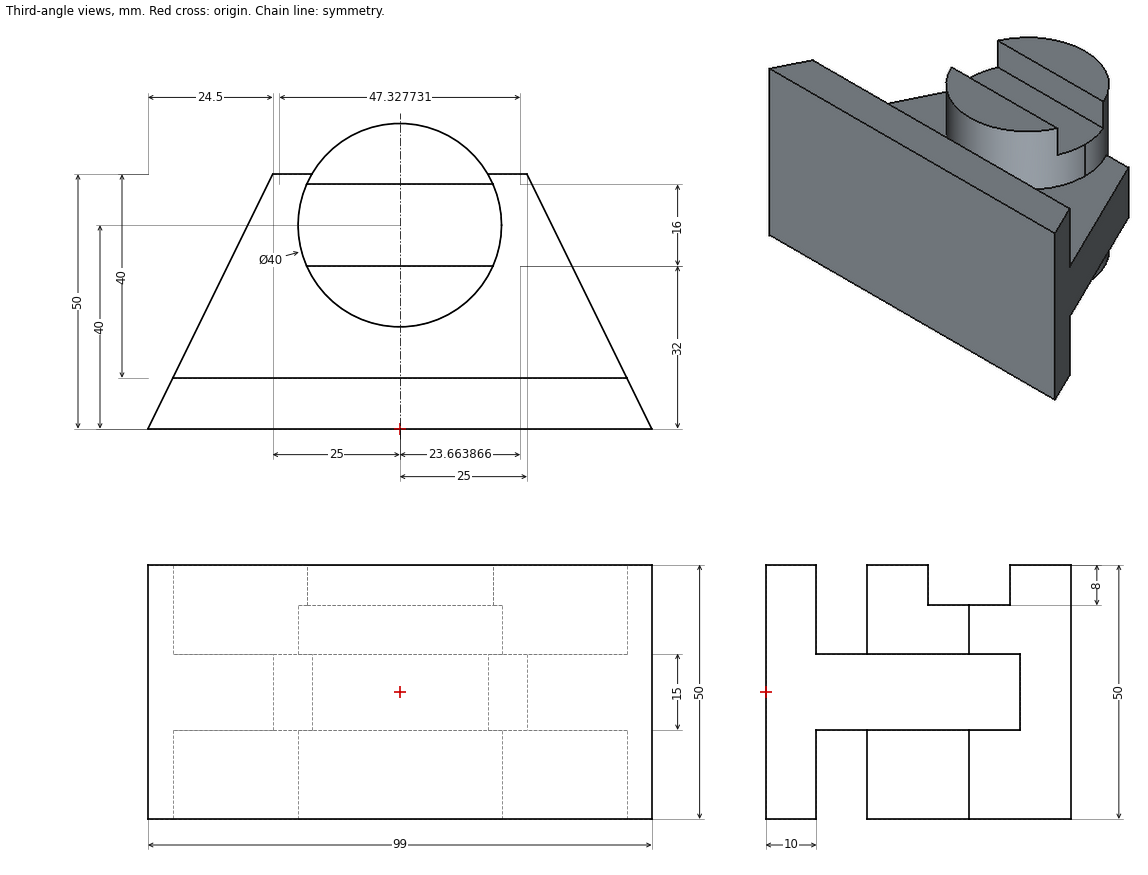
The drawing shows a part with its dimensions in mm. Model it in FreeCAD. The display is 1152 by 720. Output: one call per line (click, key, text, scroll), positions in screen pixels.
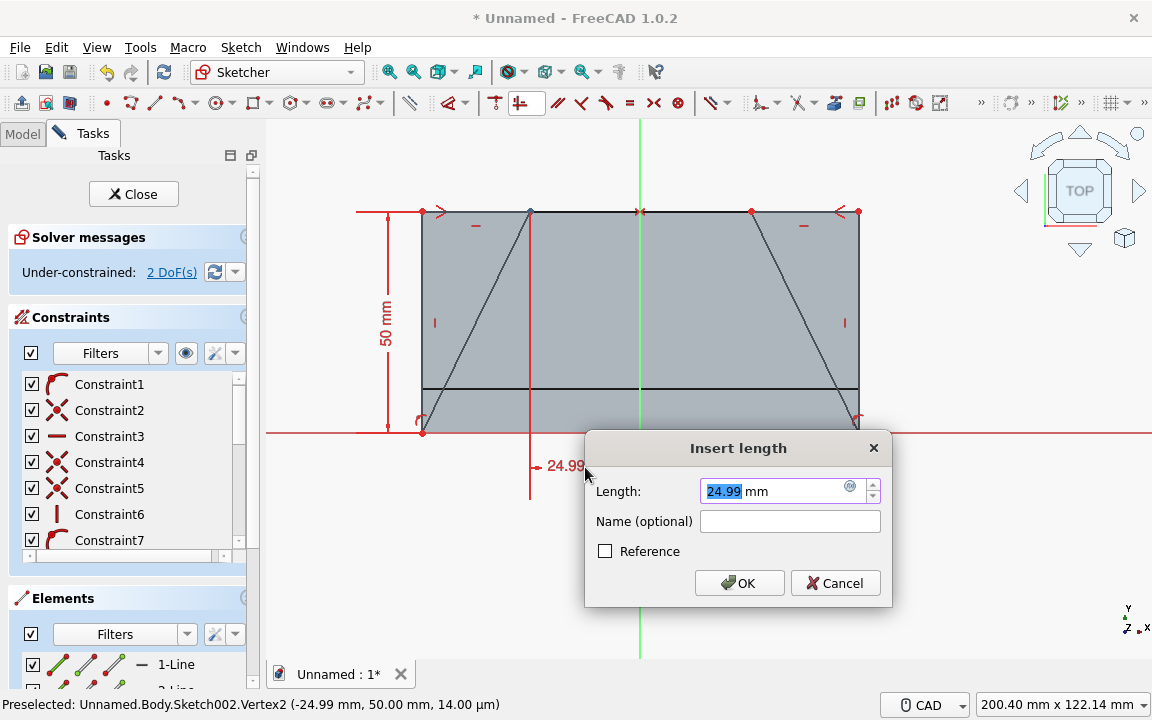
text(25)
key(Return)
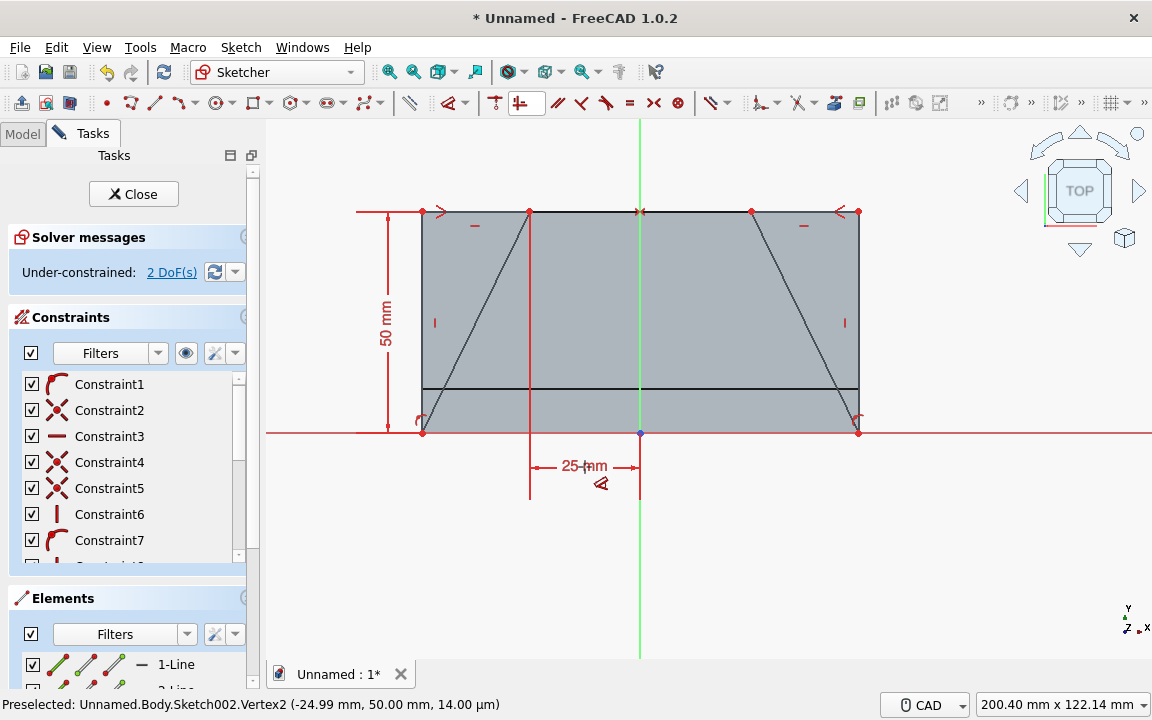
click(751, 212)
click(696, 467)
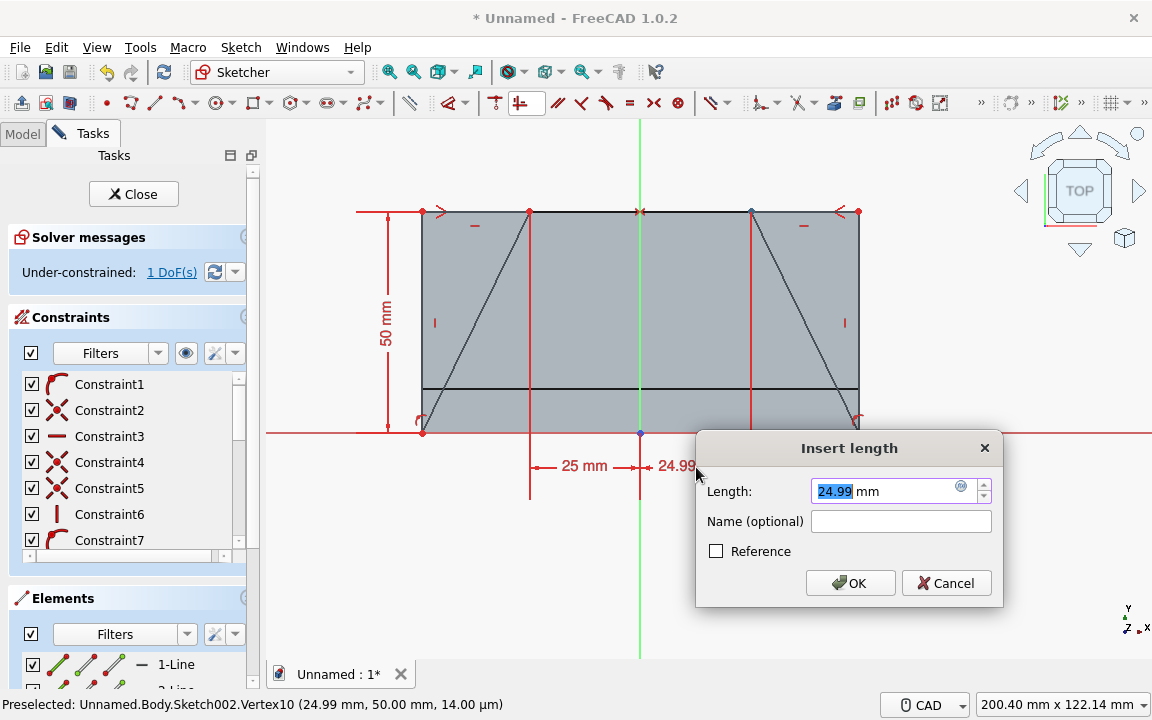
text(25)
key(Return)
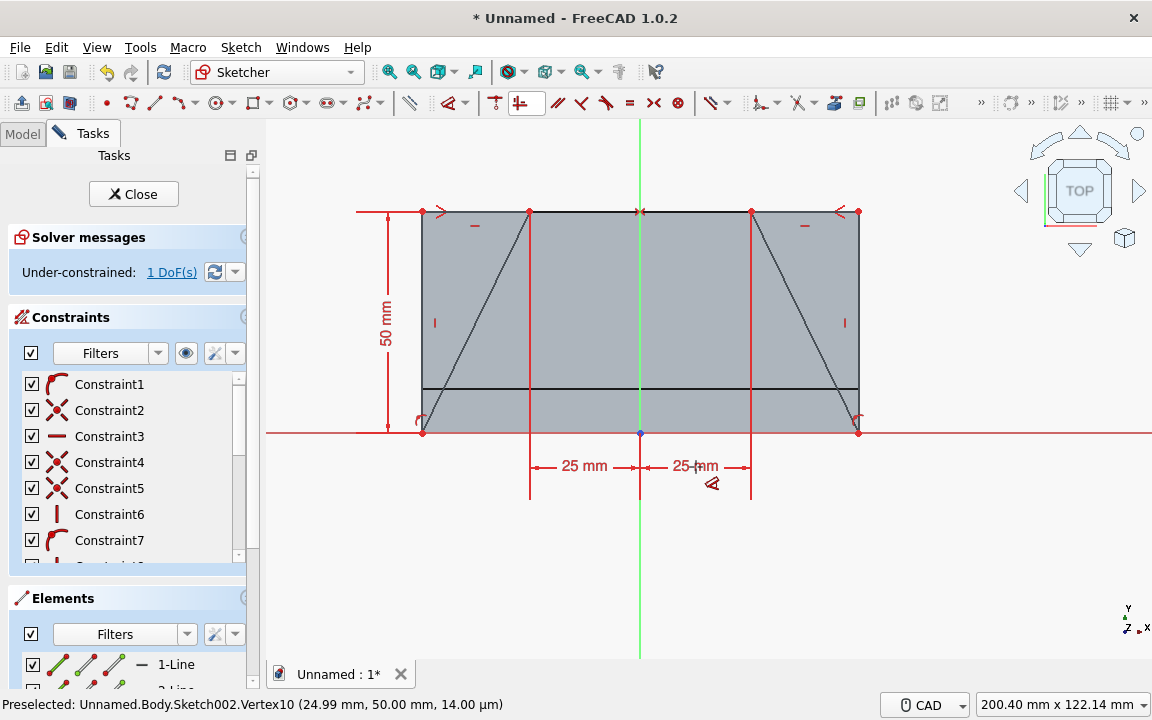
click(498, 212)
click(476, 178)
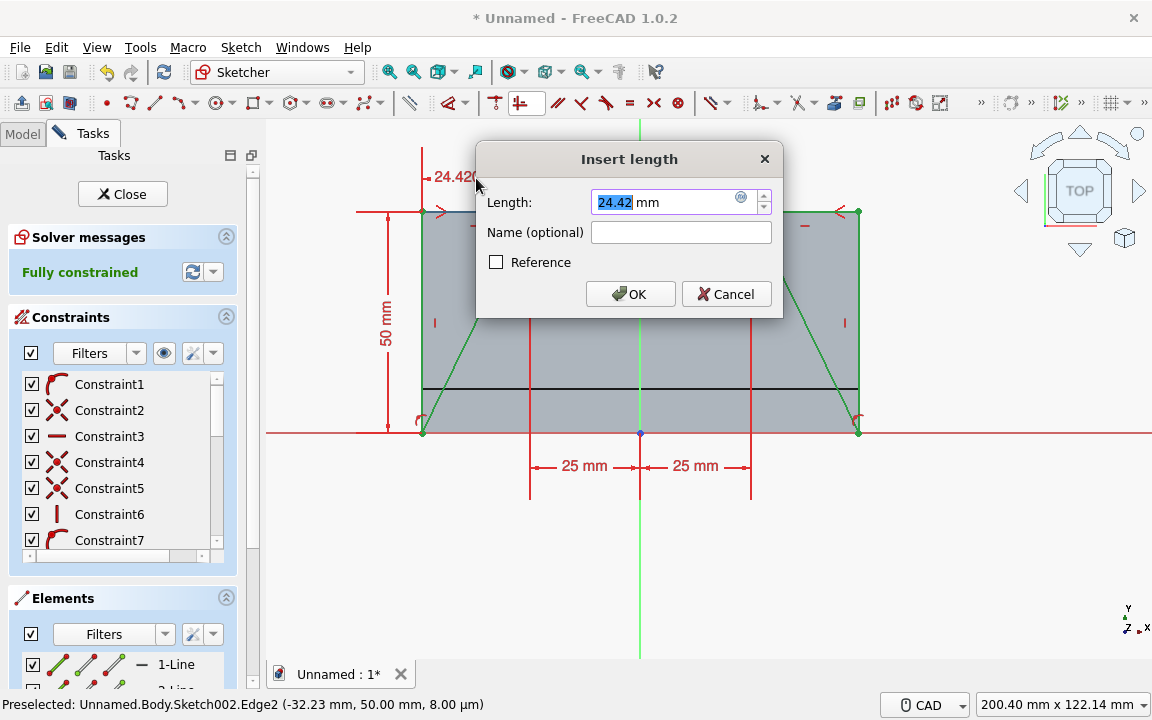
text(24.5)
key(Return)
key(Escape)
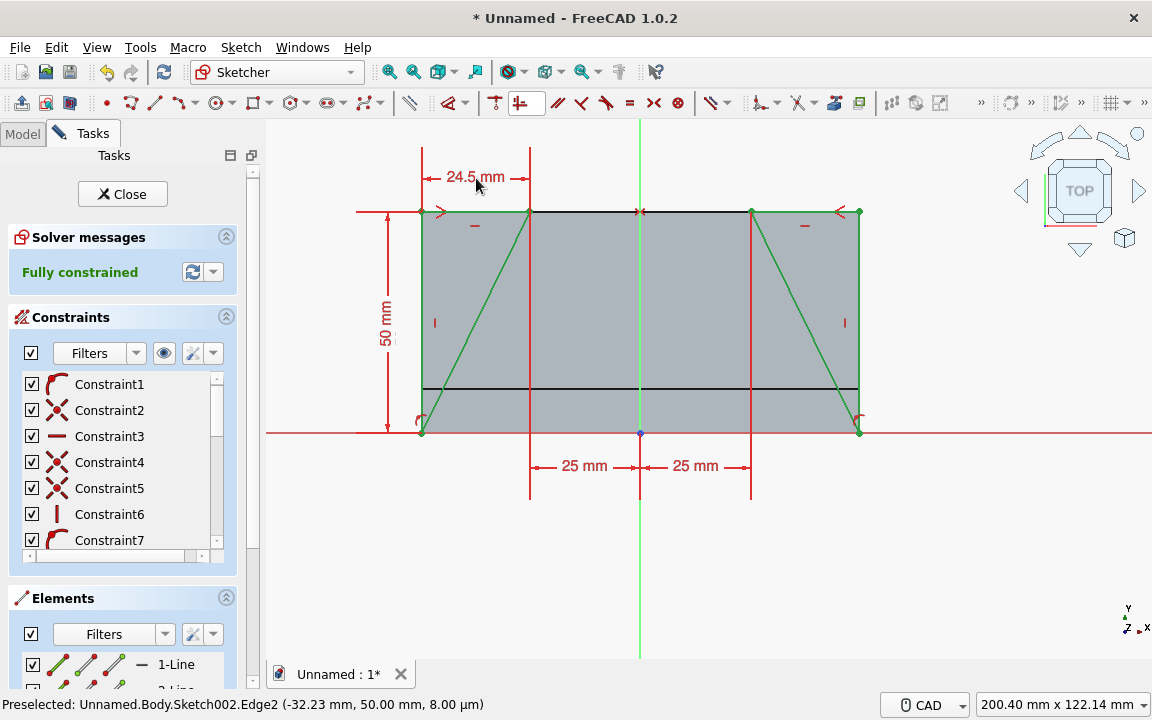
click(123, 194)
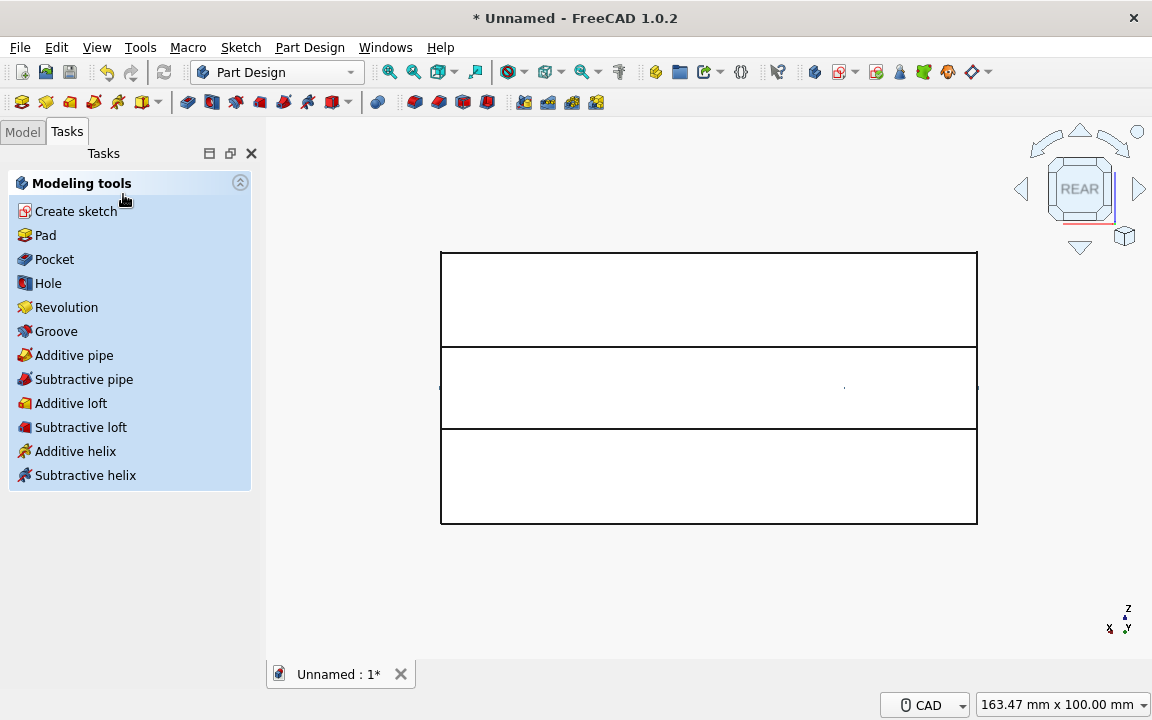
click(188, 102)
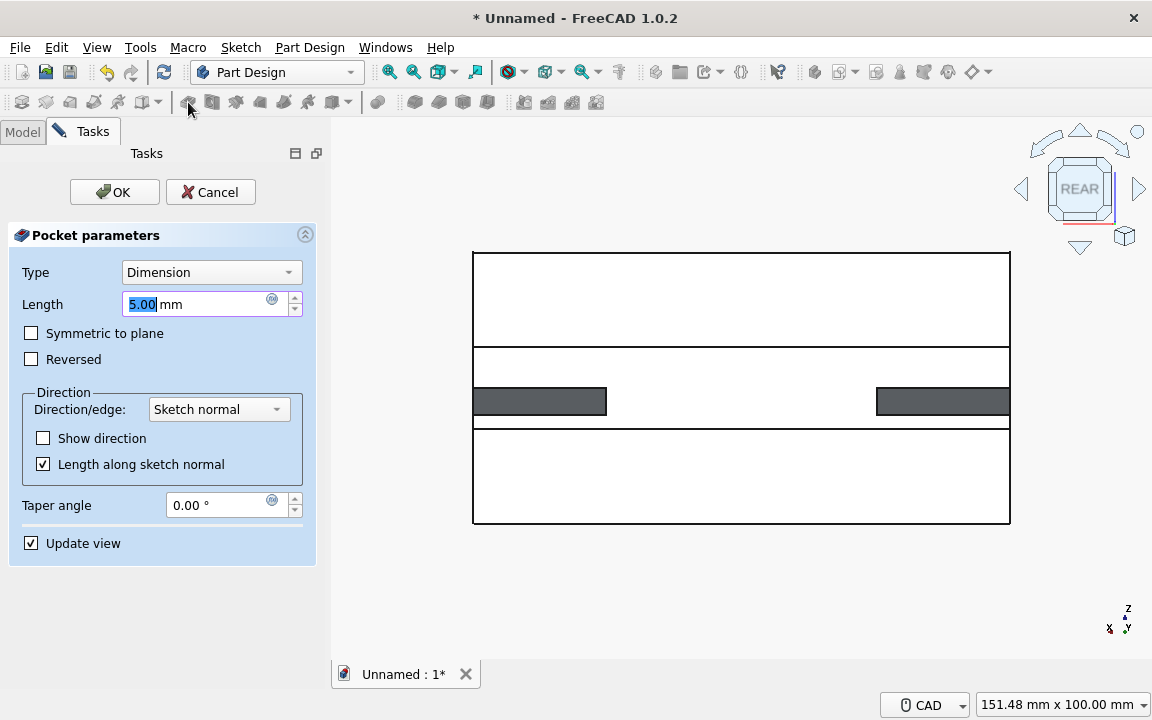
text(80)
key(Tab)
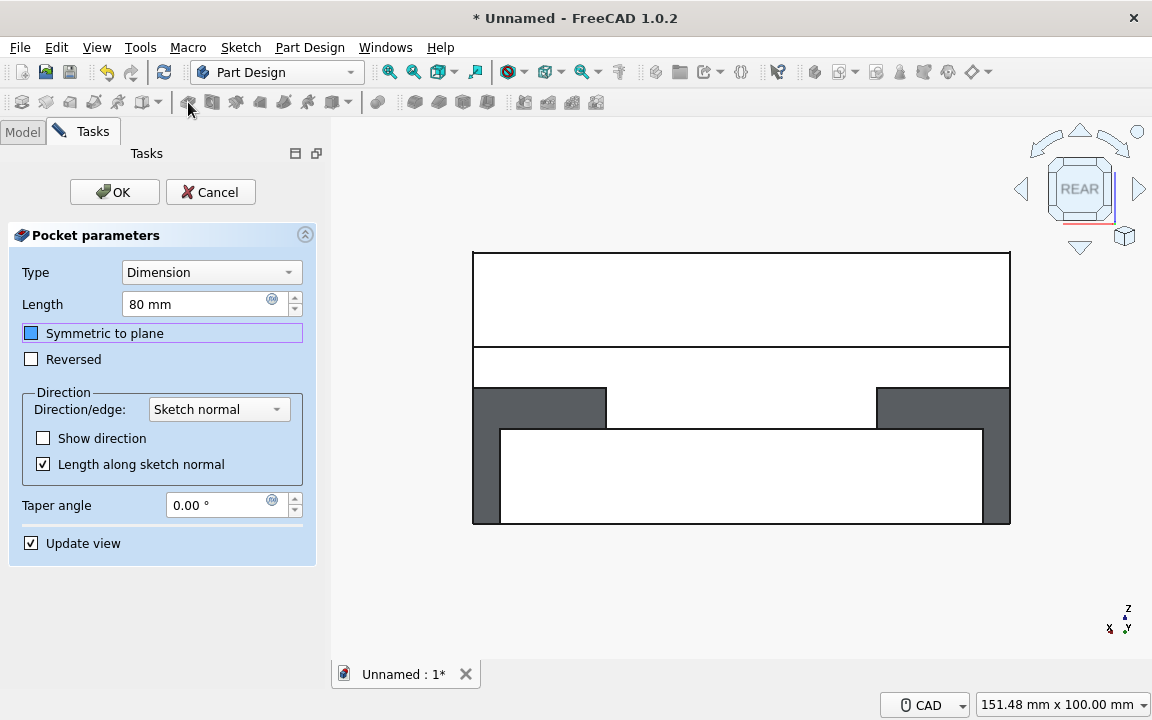
click(30, 333)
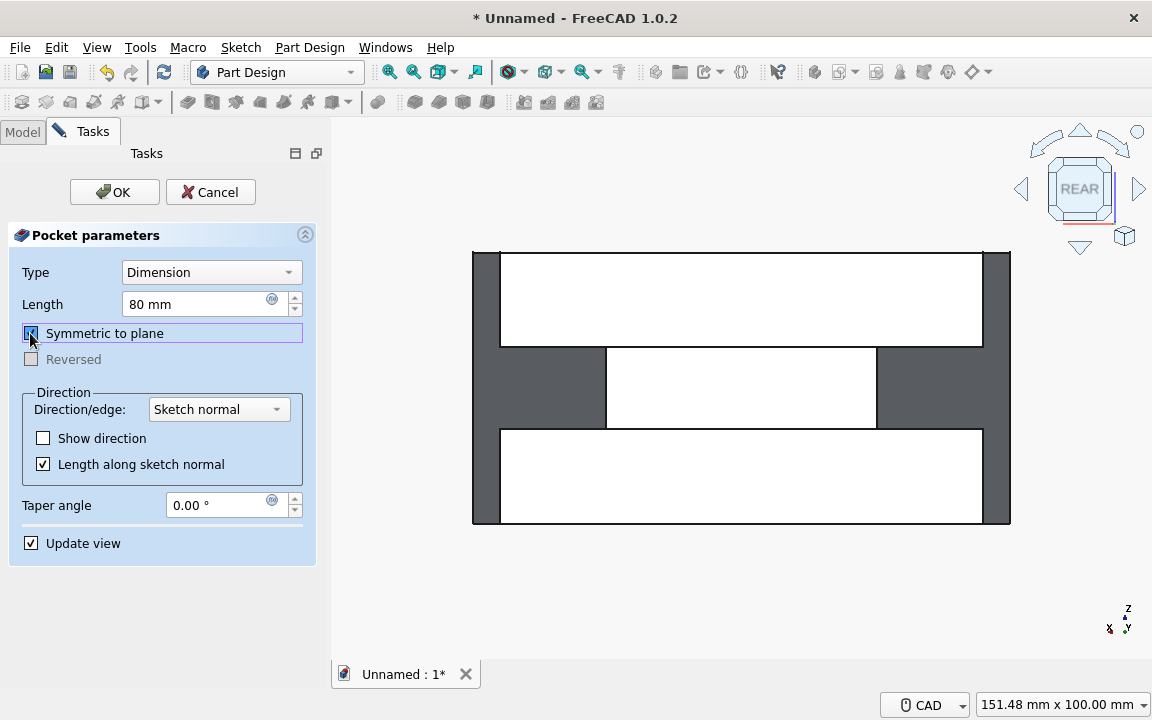
click(115, 192)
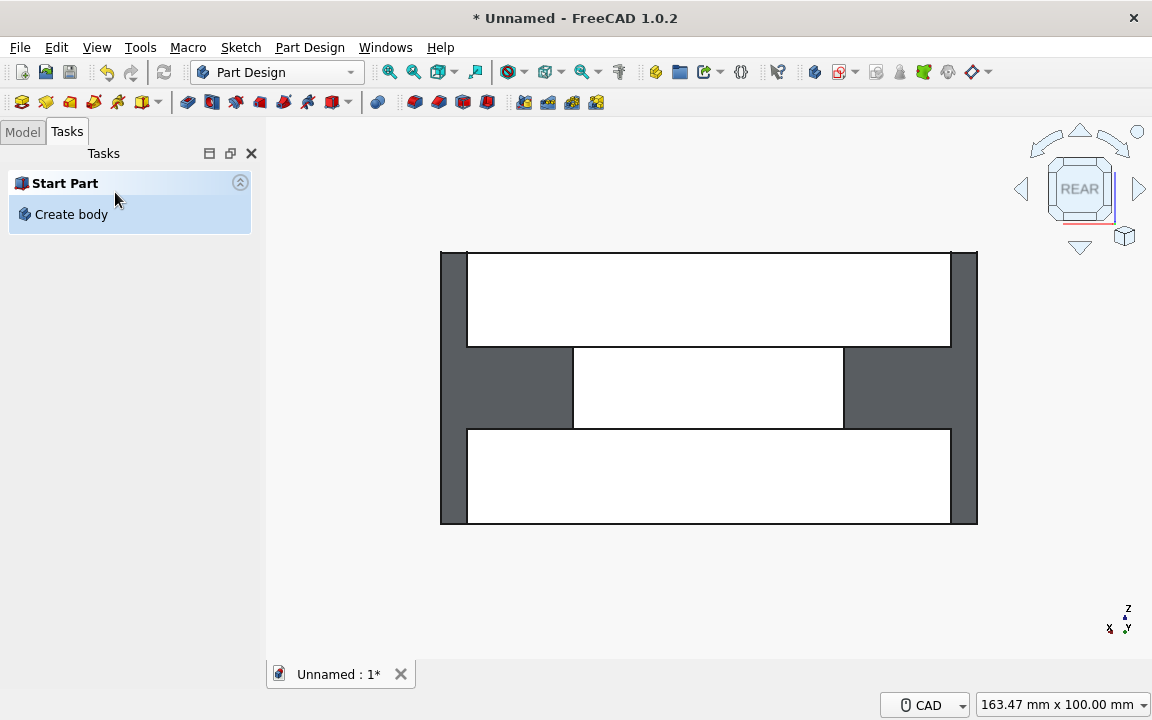
click(840, 72)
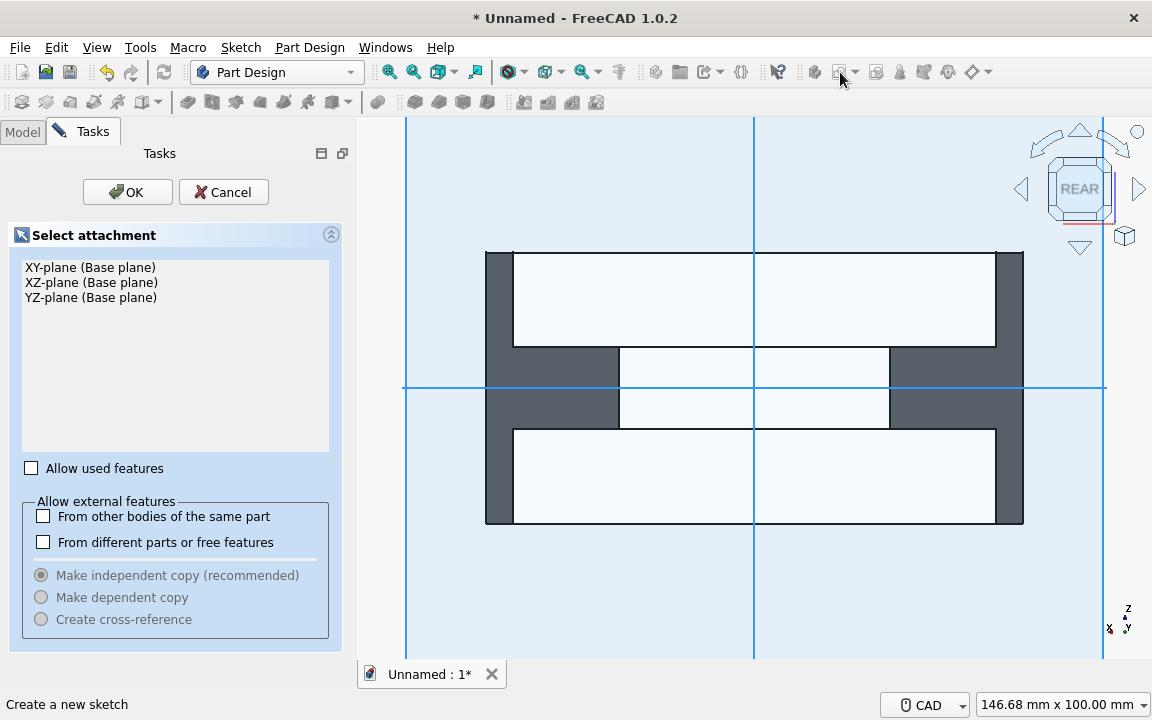
click(82, 268)